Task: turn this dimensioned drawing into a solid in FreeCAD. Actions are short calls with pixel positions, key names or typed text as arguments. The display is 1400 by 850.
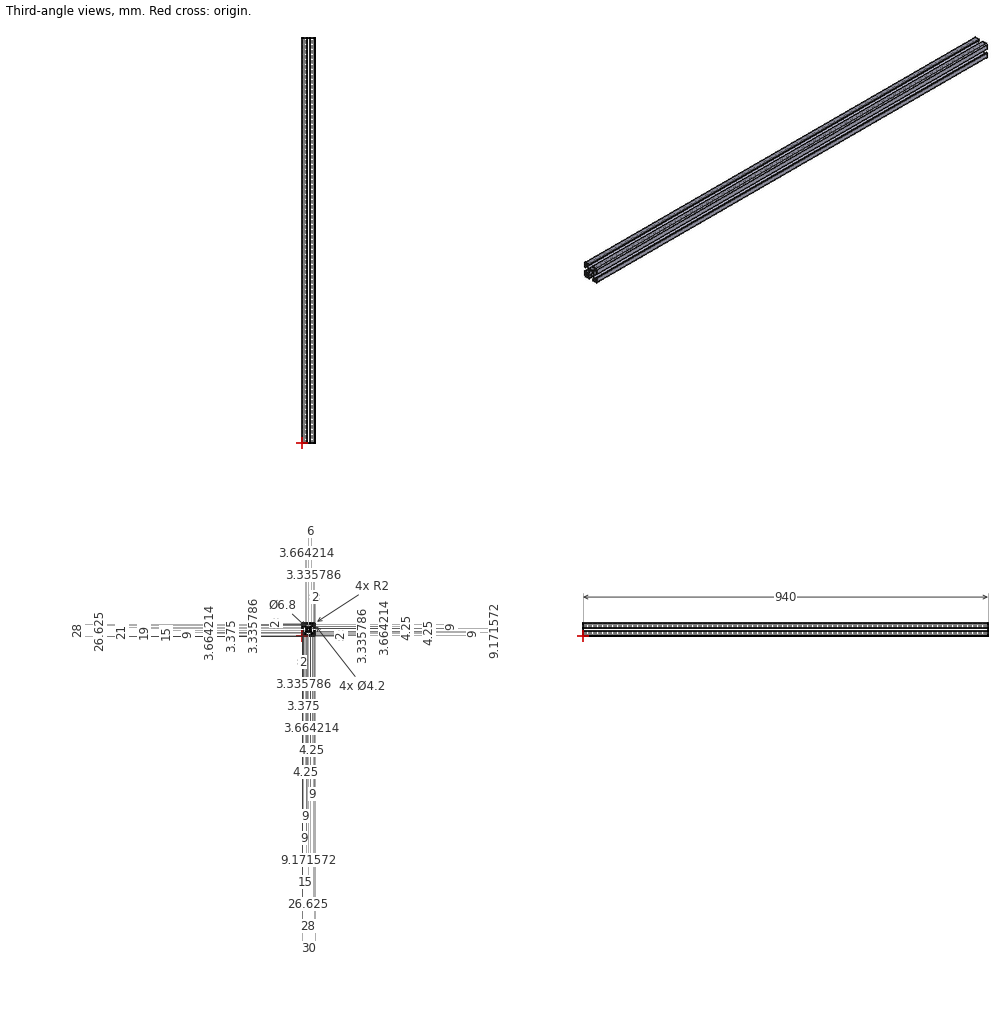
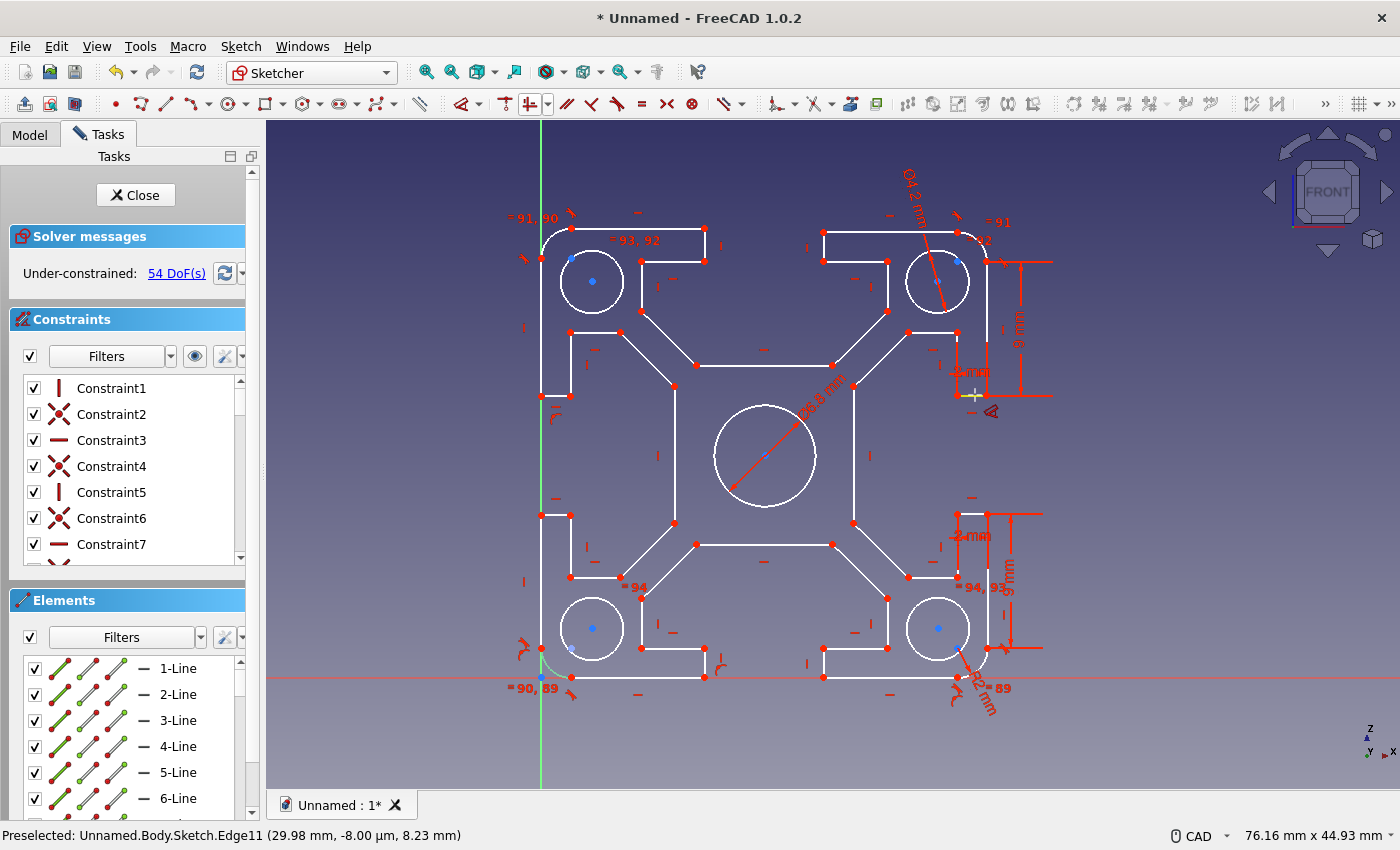
click(918, 678)
click(891, 712)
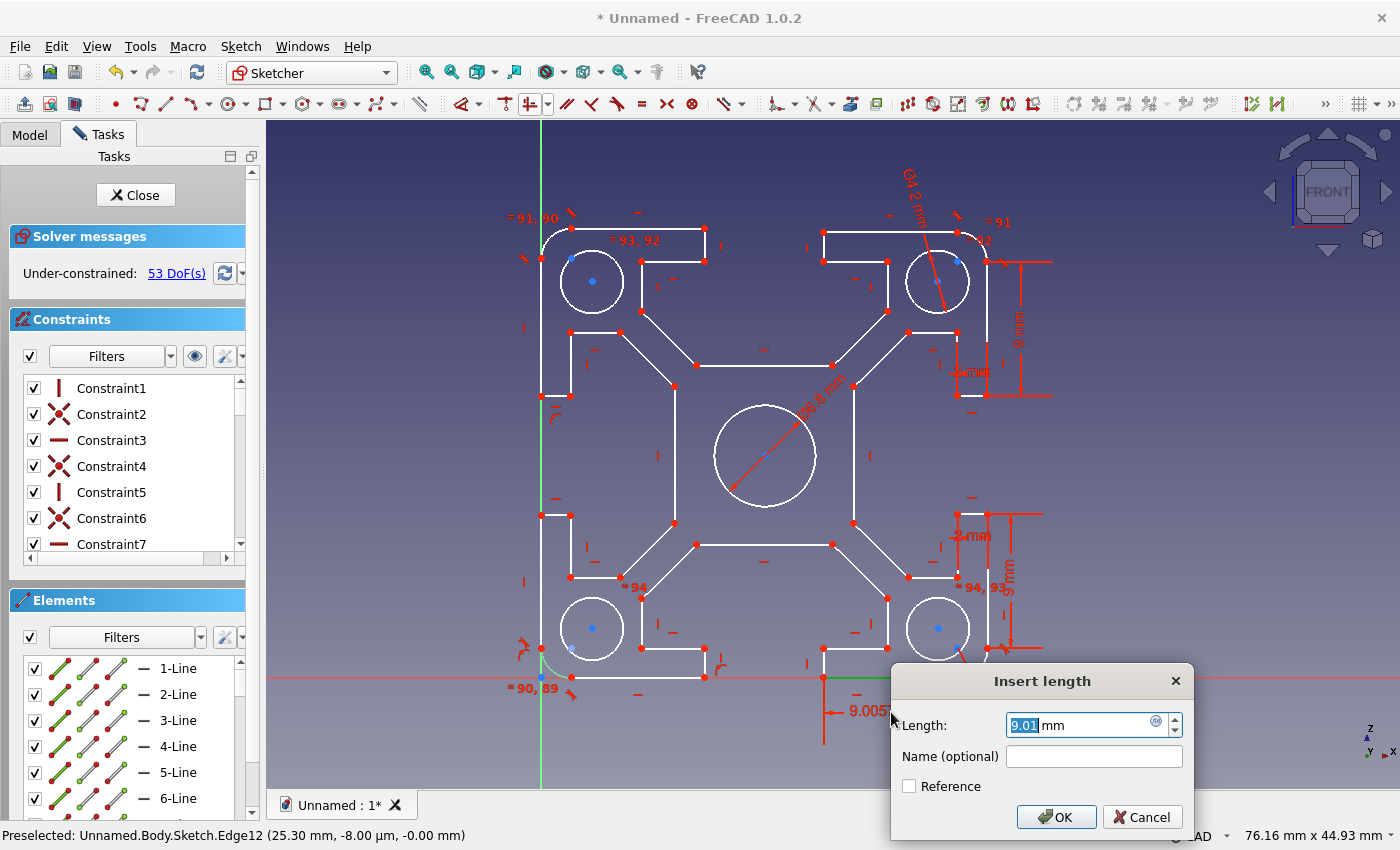
text(9)
key(Return)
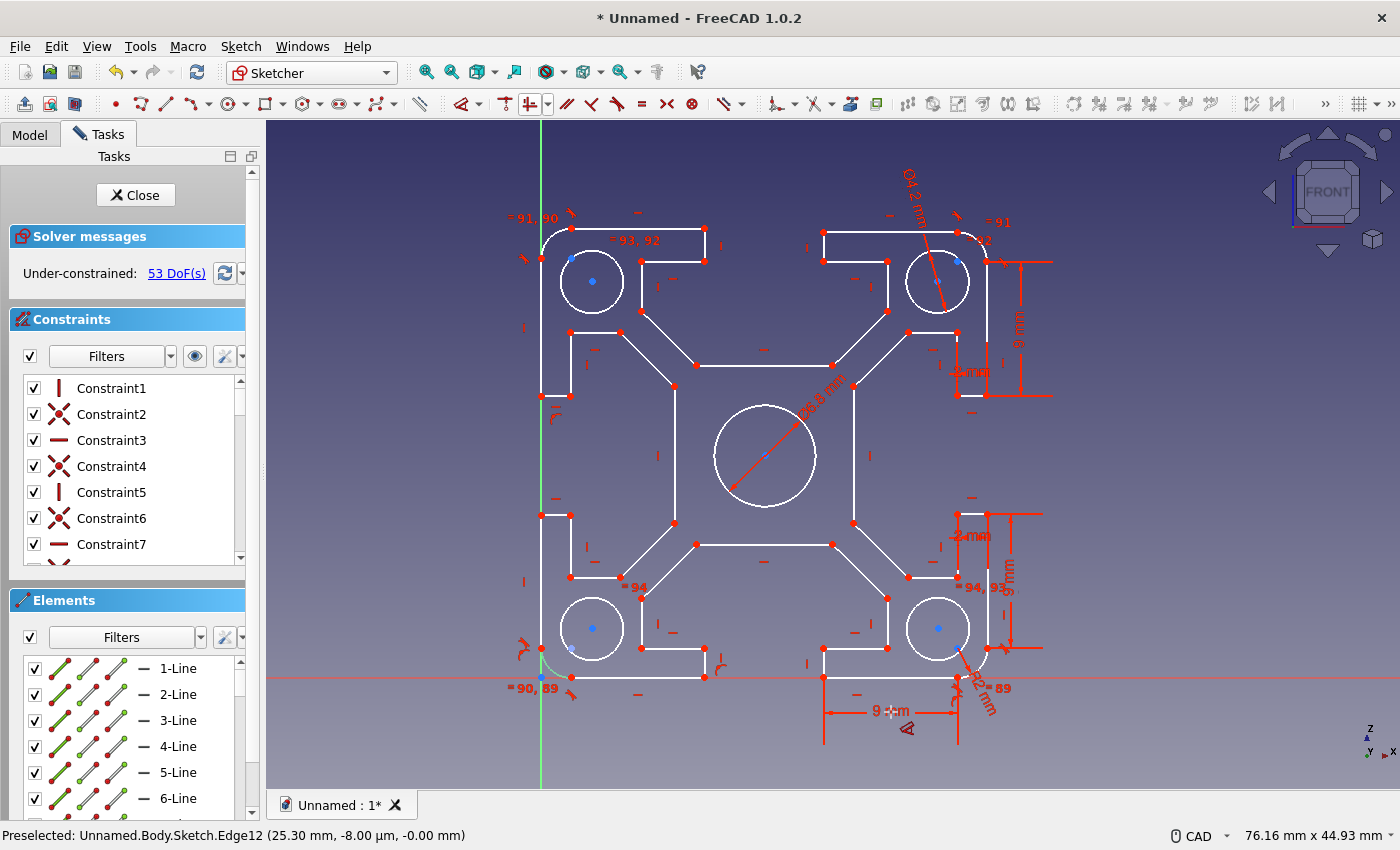
scroll(824, 666, up, 2)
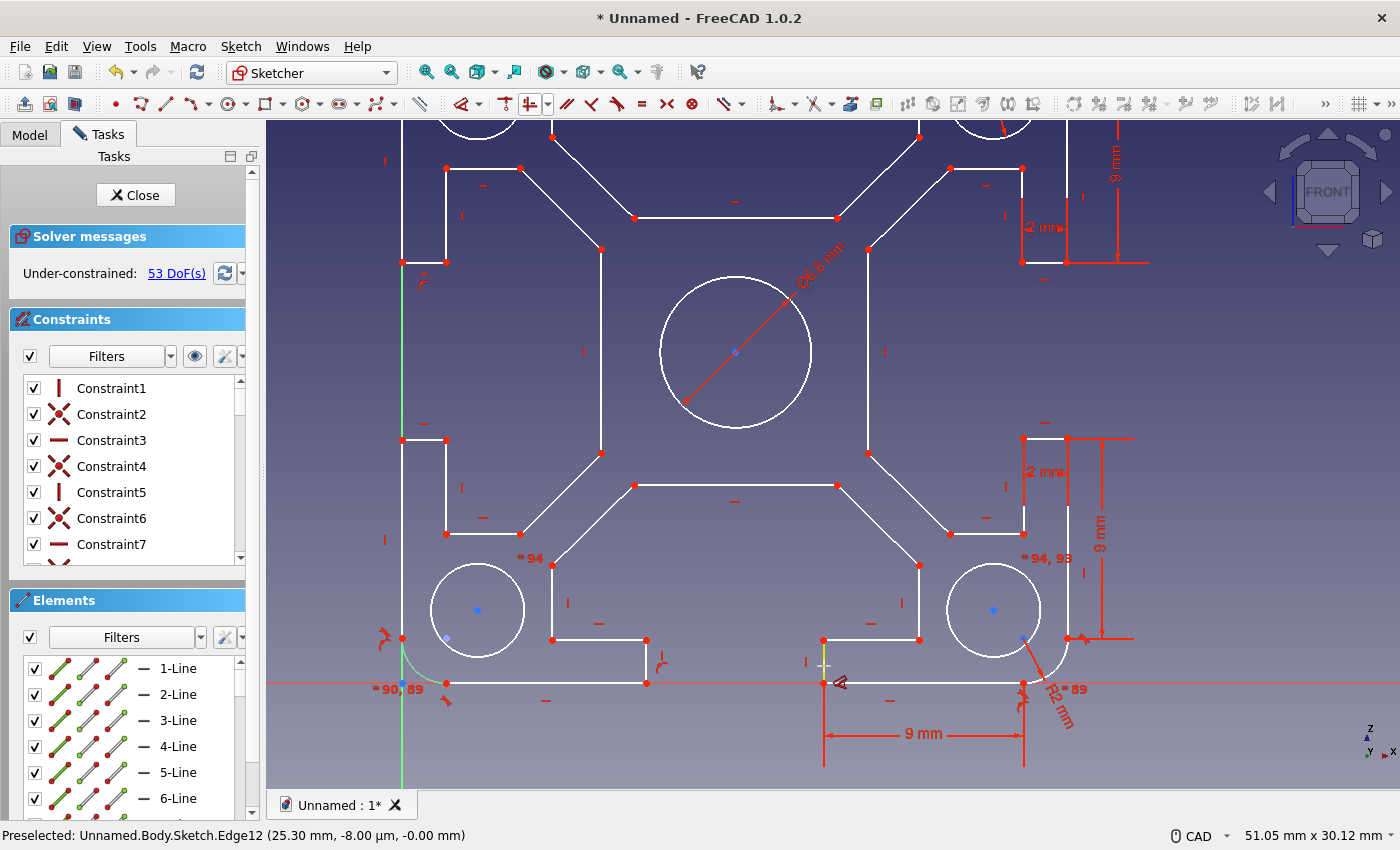
click(824, 666)
click(858, 662)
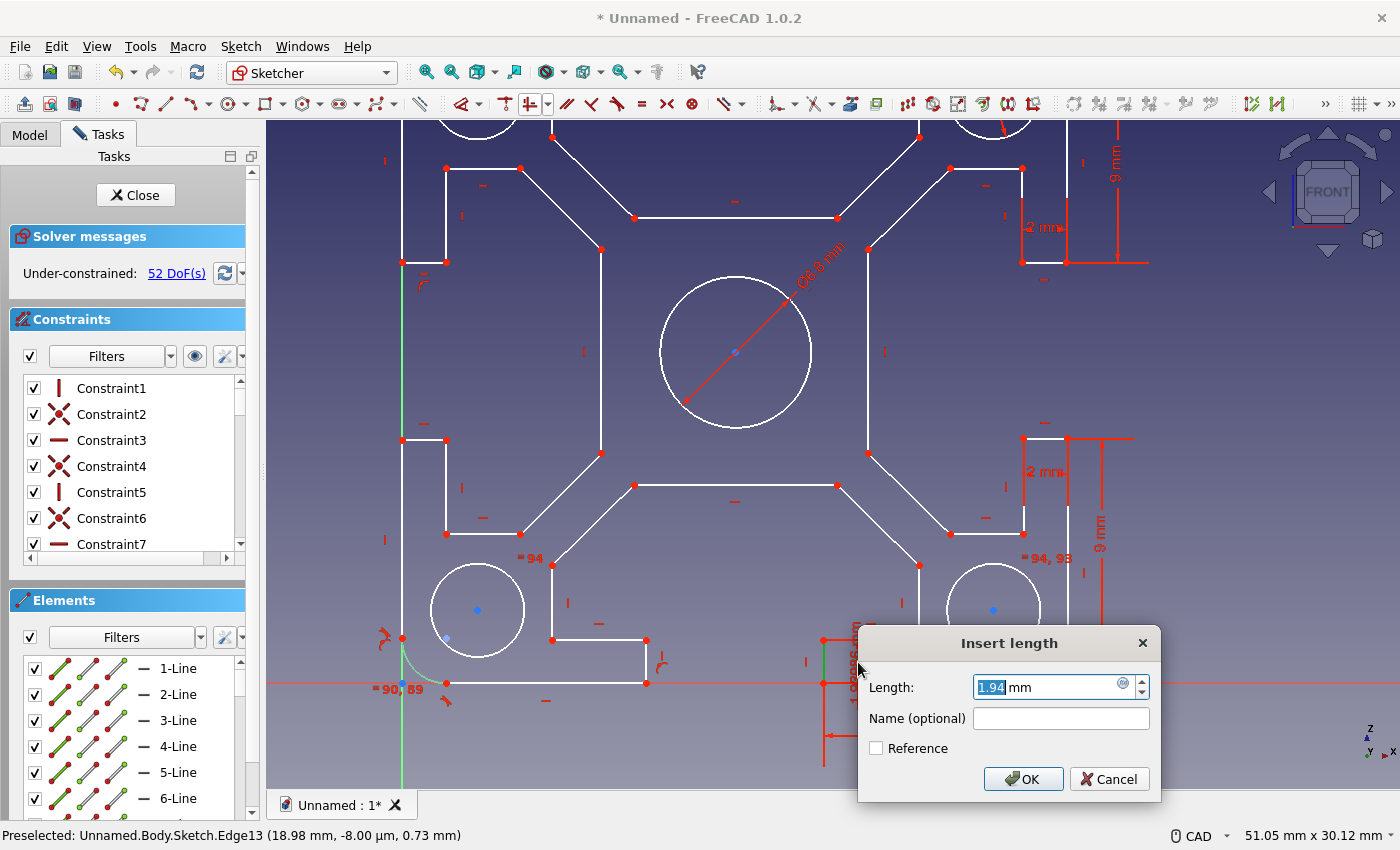
text(2)
key(Return)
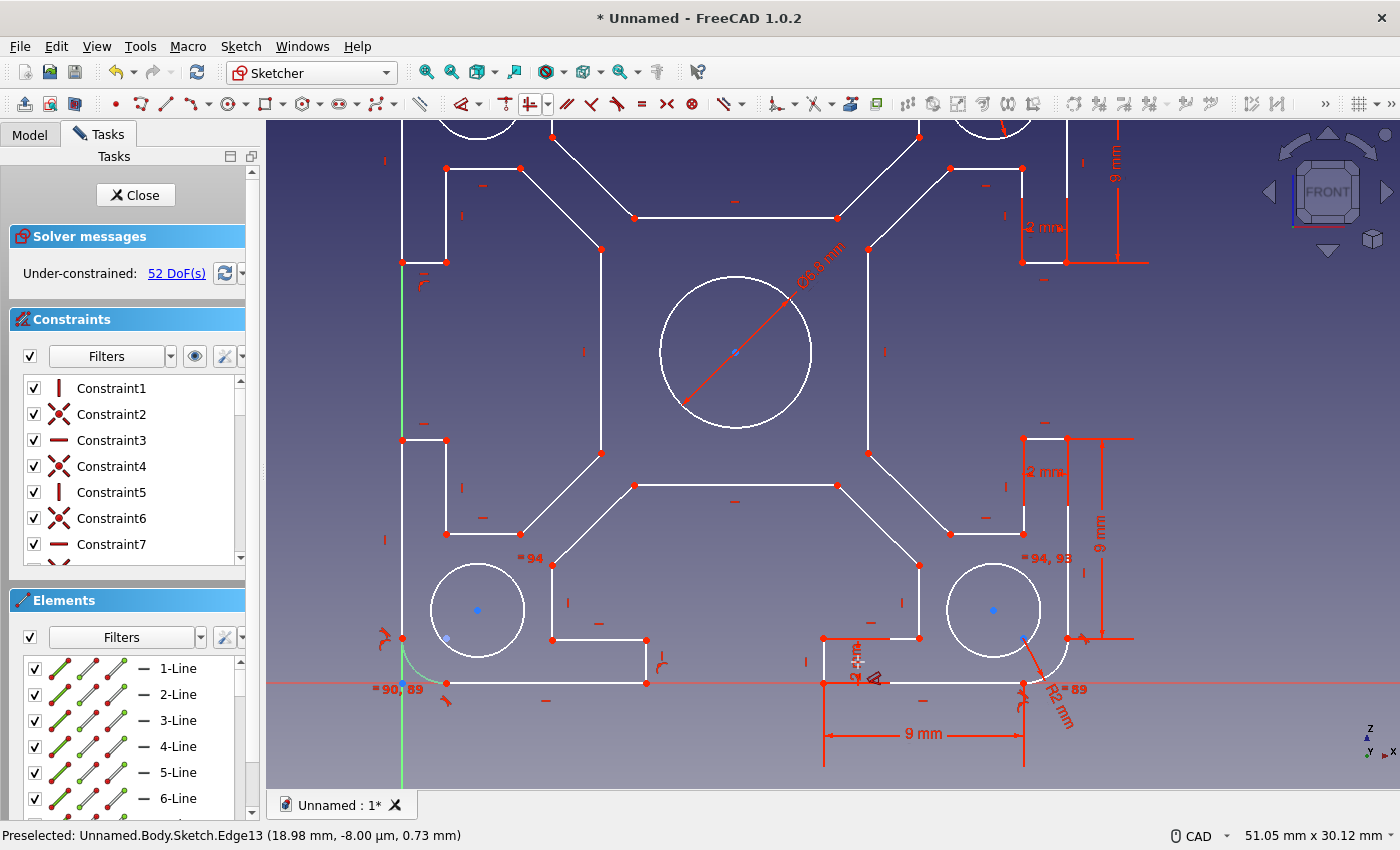
click(646, 653)
click(612, 662)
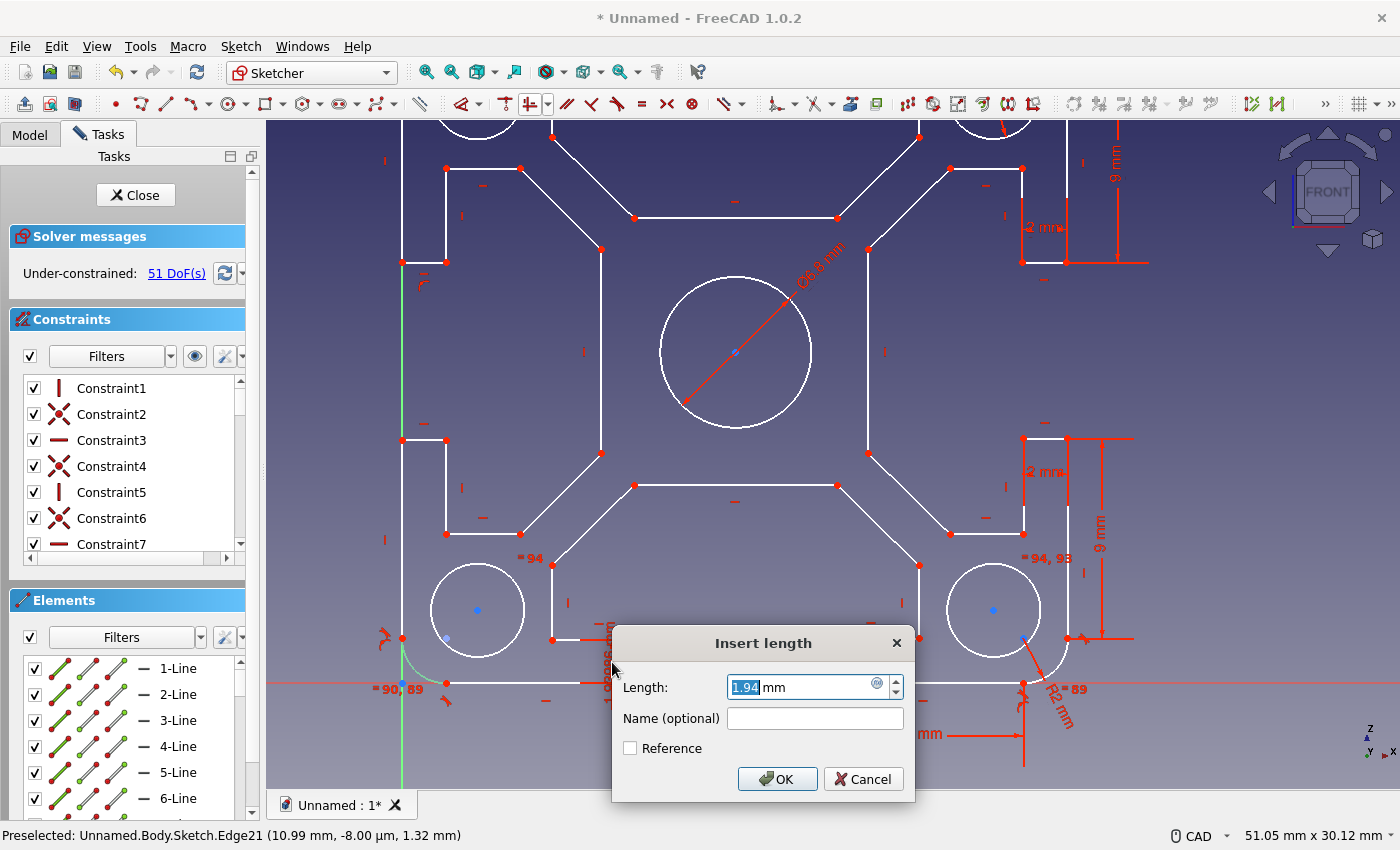
text(2)
key(Return)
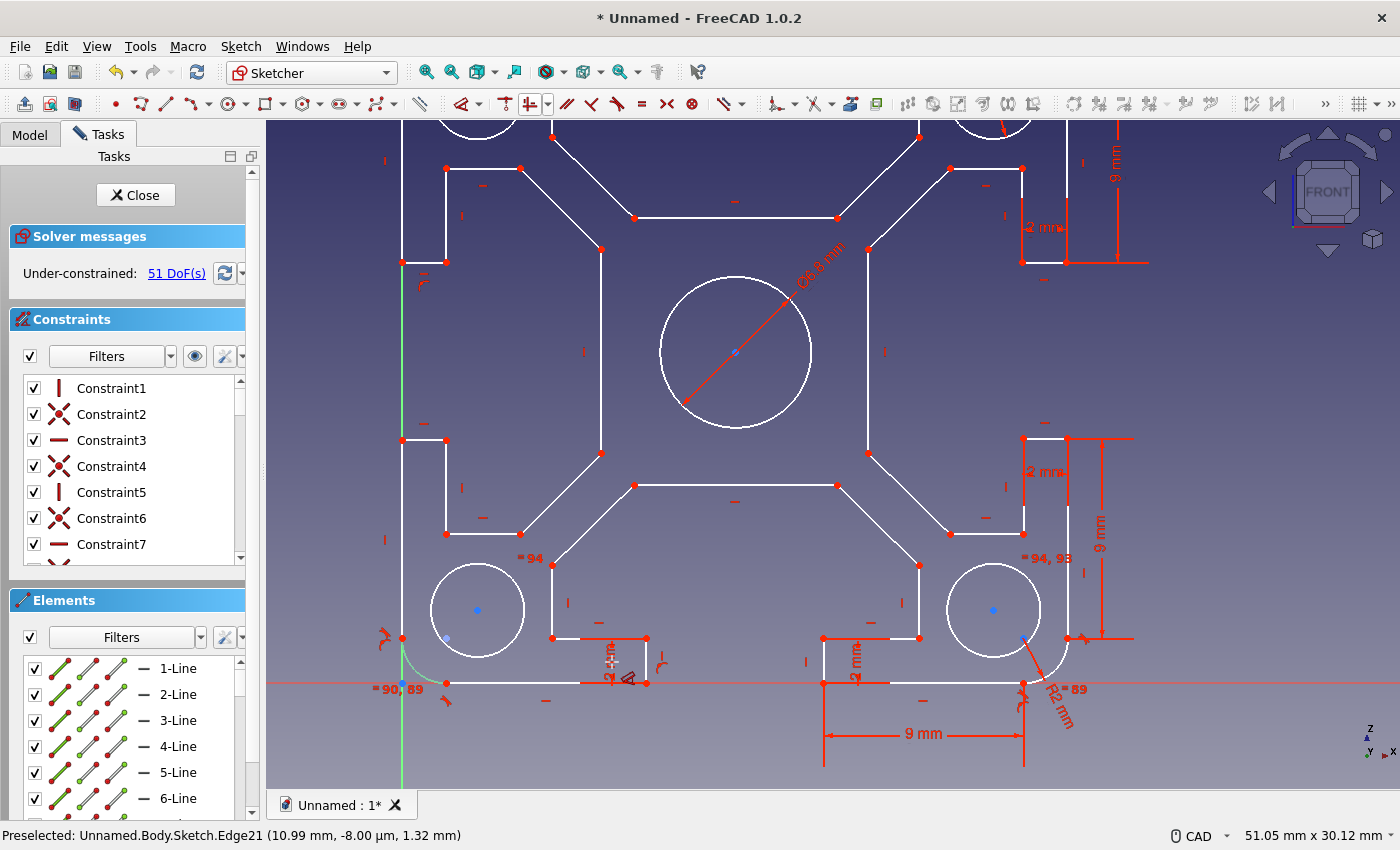
click(586, 683)
click(546, 717)